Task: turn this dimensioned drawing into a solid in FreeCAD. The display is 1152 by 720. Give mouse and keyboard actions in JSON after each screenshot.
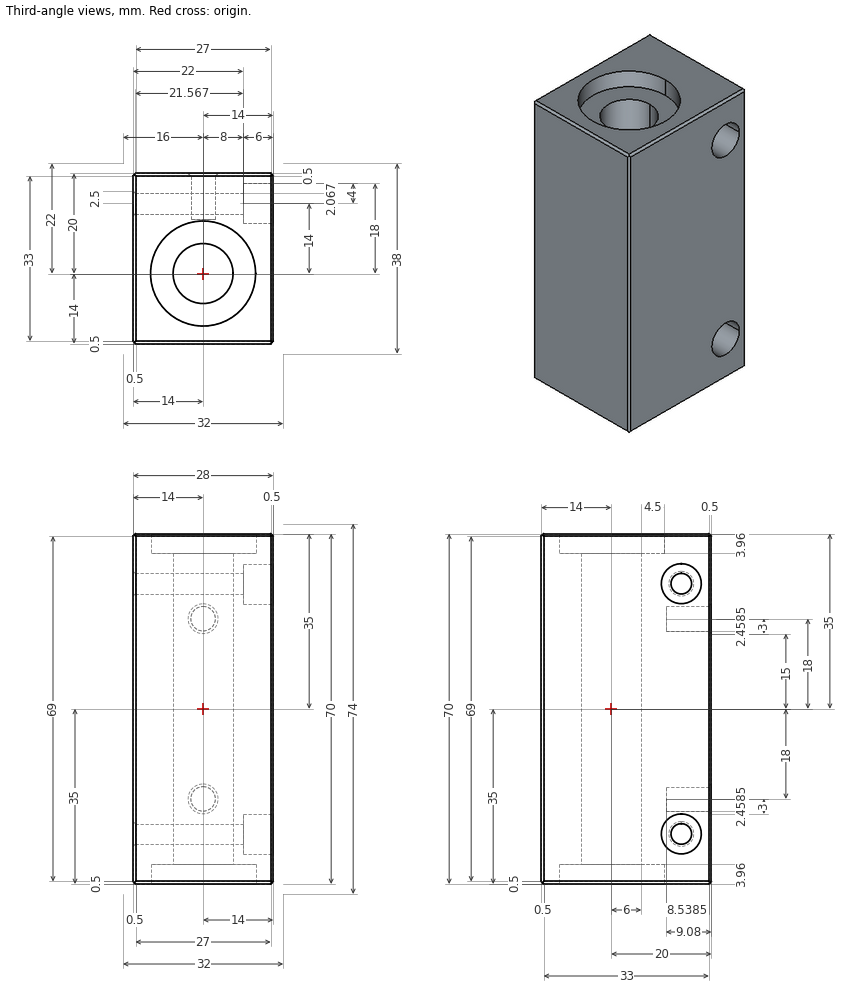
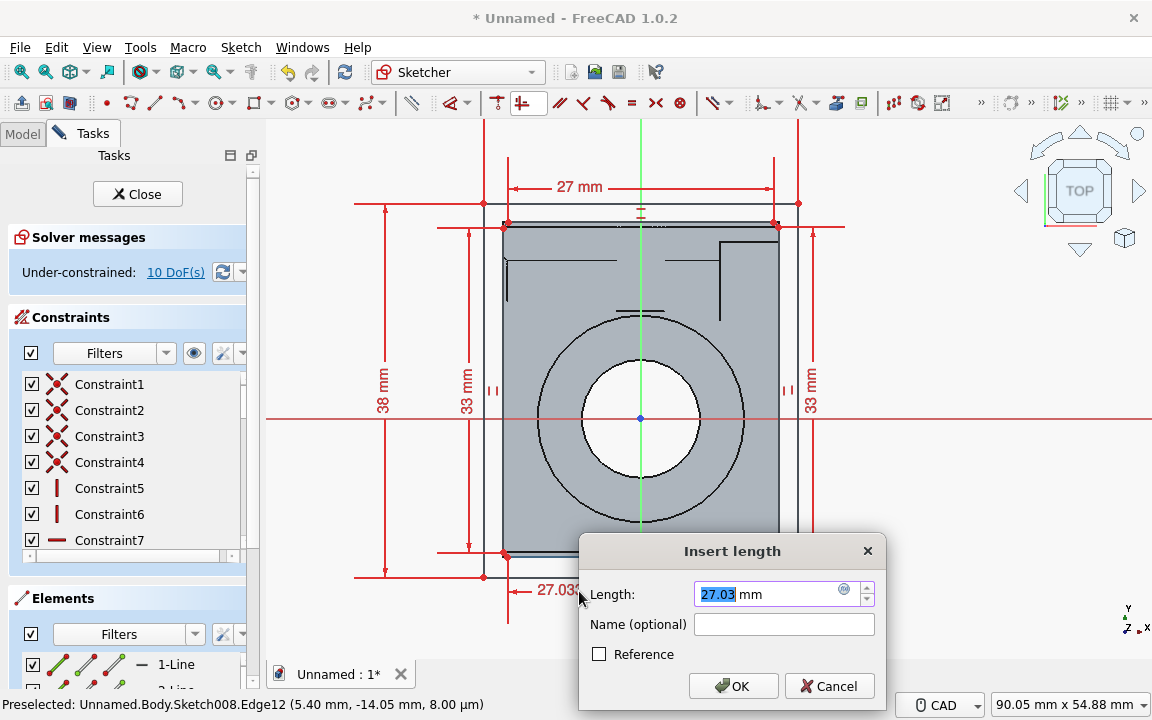
{"action": "type", "text": "27"}
{"action": "key", "text": "Return"}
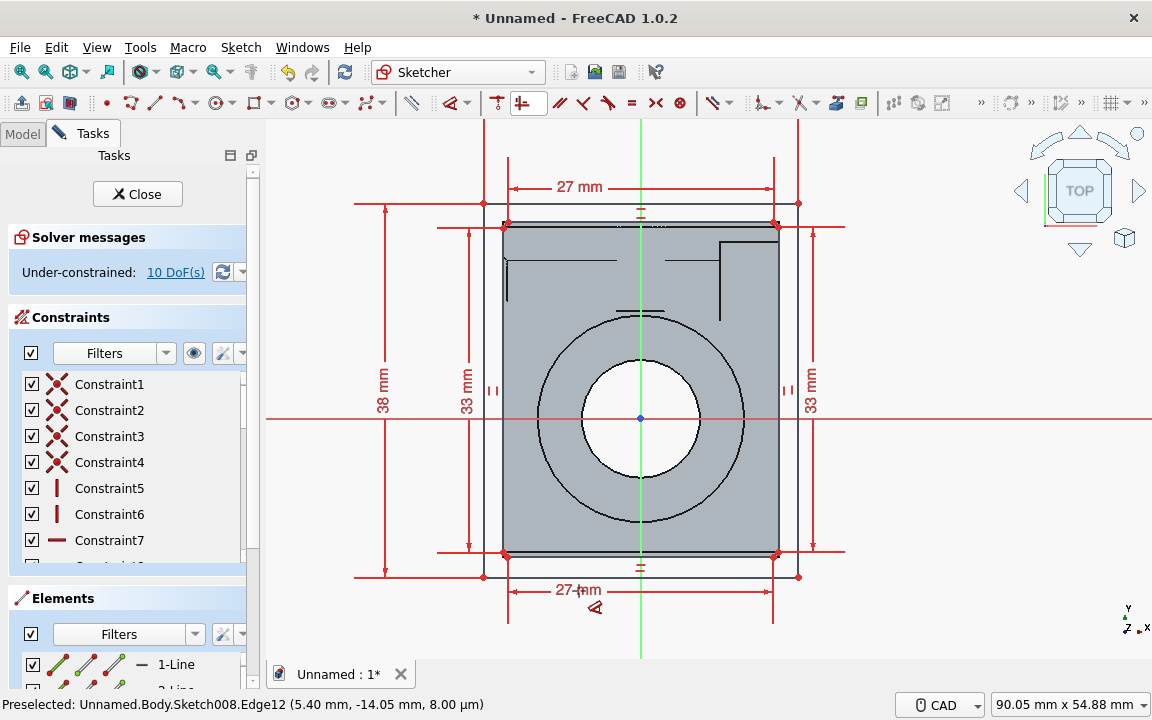
{"action": "left_click", "coordinate": [484, 204]}
{"action": "left_click", "coordinate": [507, 170]}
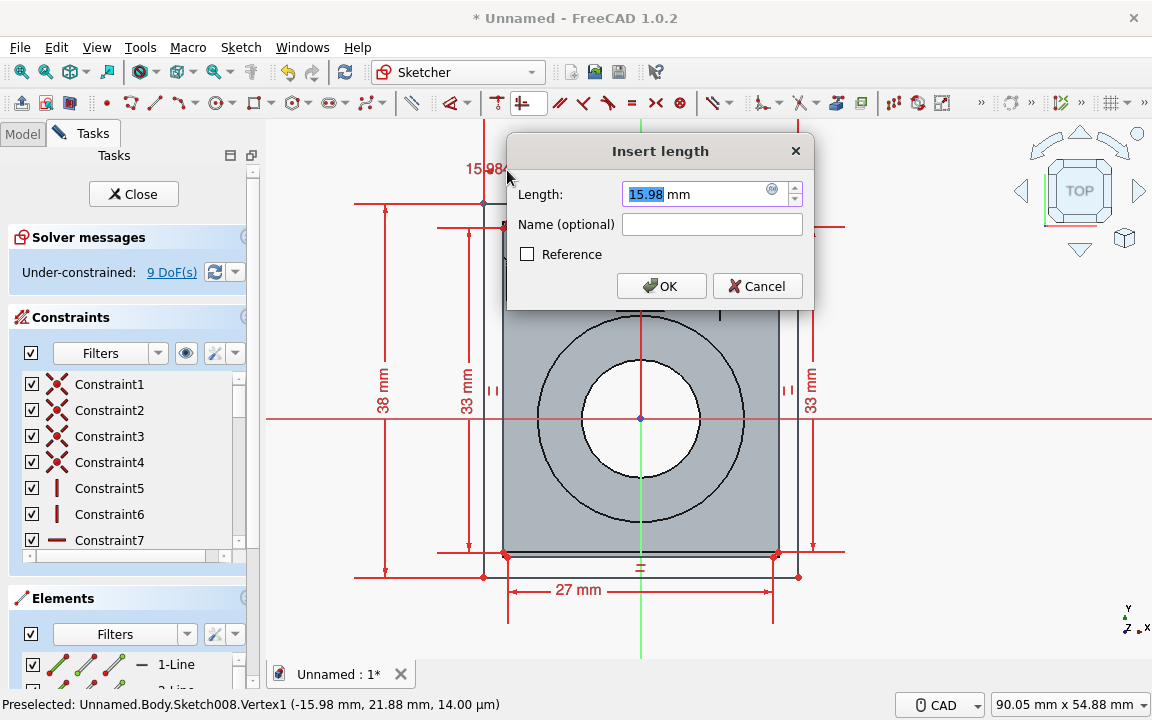
{"action": "type", "text": "16"}
{"action": "key", "text": "Return"}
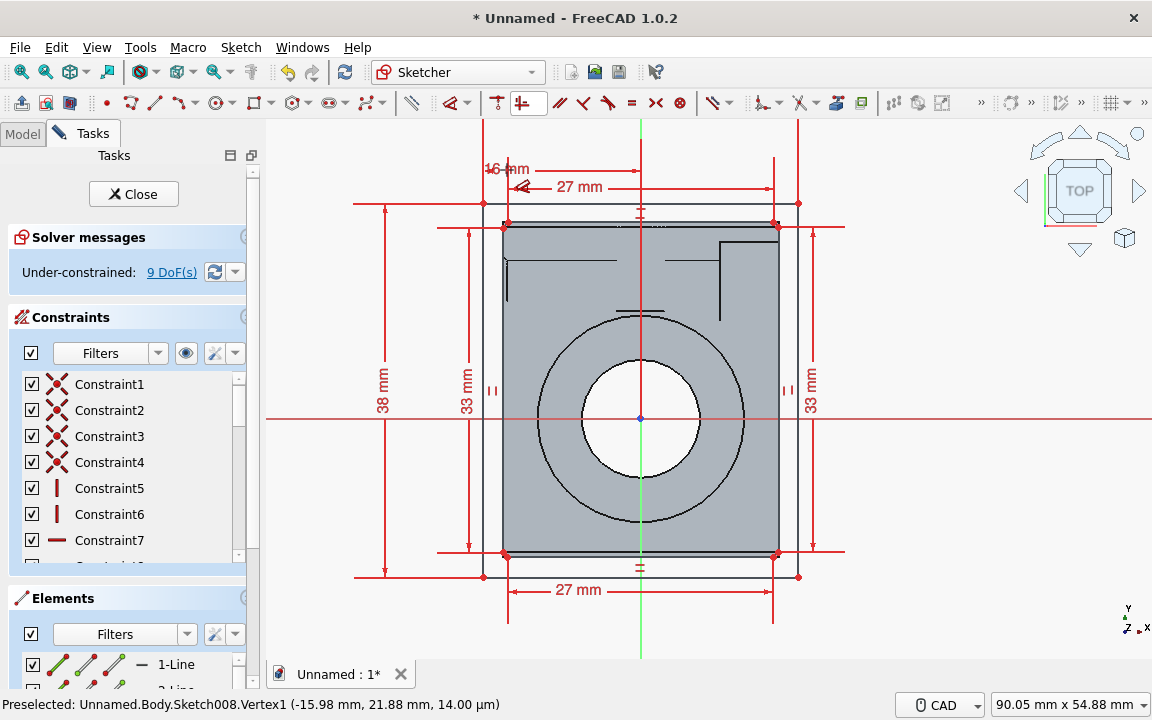
{"action": "left_click", "coordinate": [483, 204]}
{"action": "left_click", "coordinate": [449, 311]}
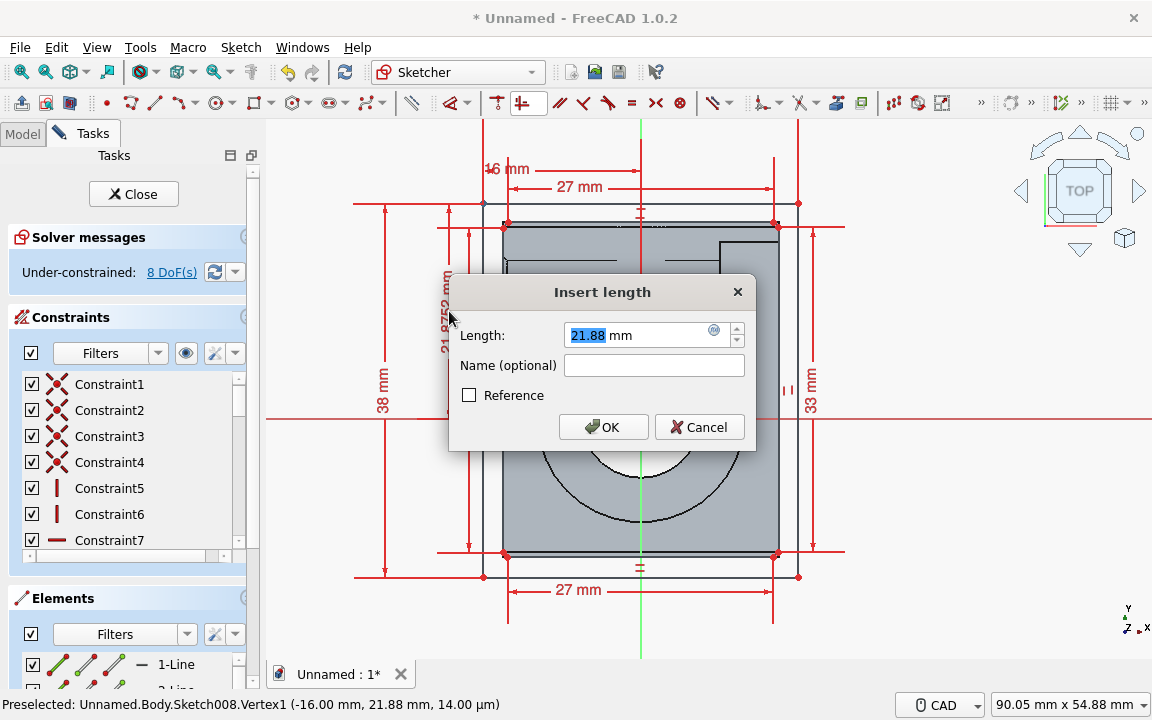
{"action": "type", "text": "22"}
{"action": "key", "text": "Return"}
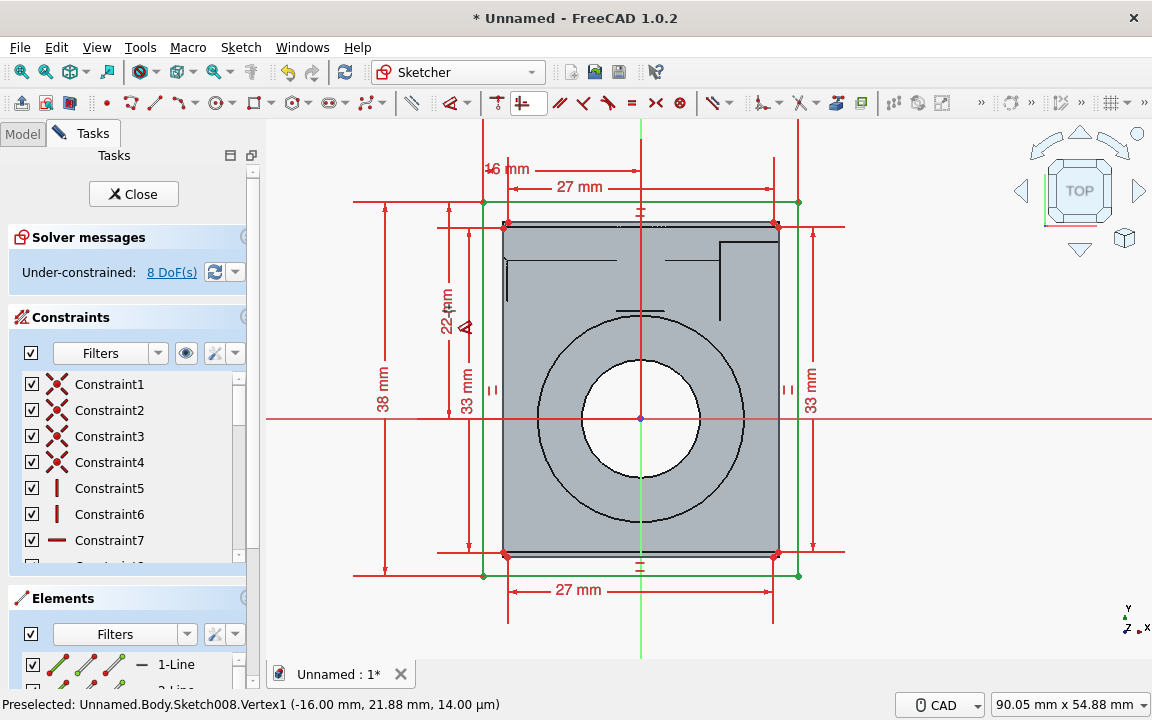
{"action": "scroll", "coordinate": [508, 557], "scroll_direction": "up", "scroll_amount": 4}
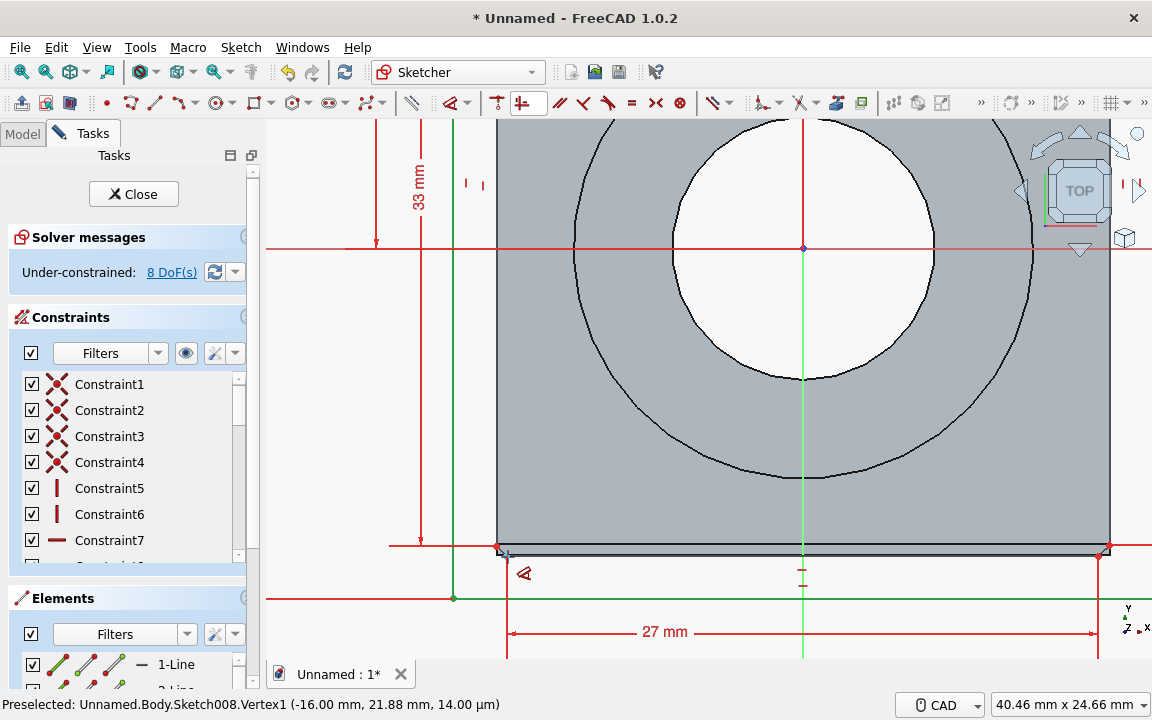
{"action": "left_click", "coordinate": [507, 556]}
{"action": "left_click", "coordinate": [473, 402]}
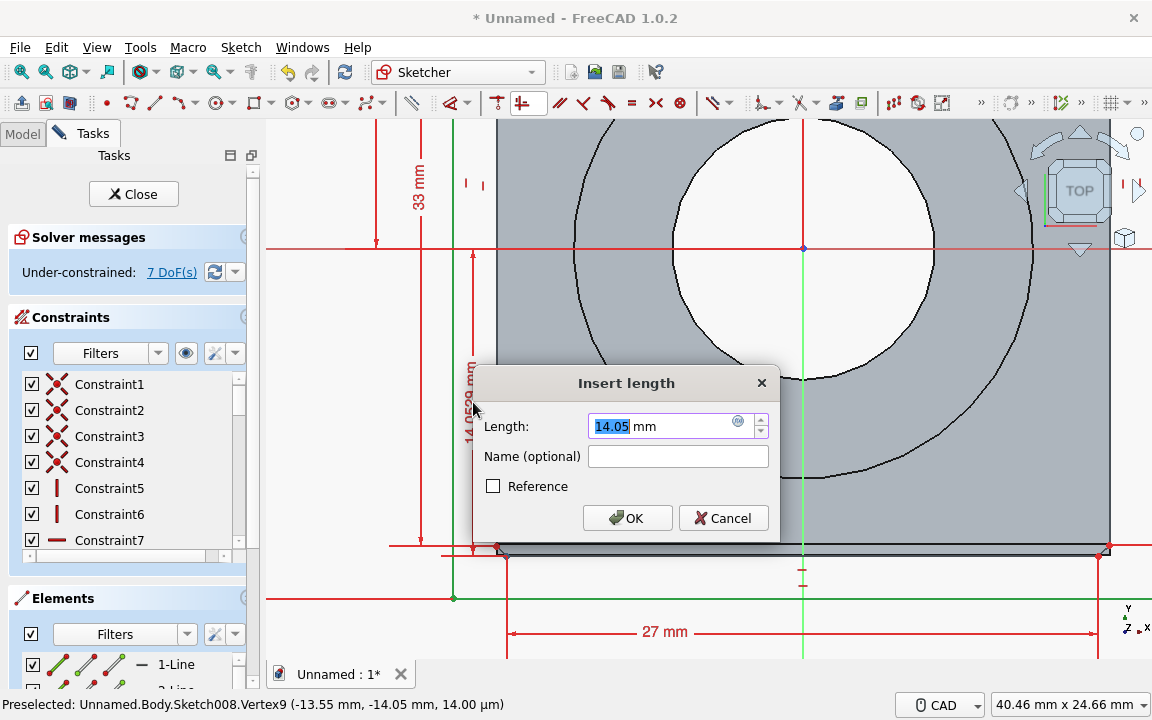
{"action": "type", "text": "14"}
{"action": "key", "text": "Return"}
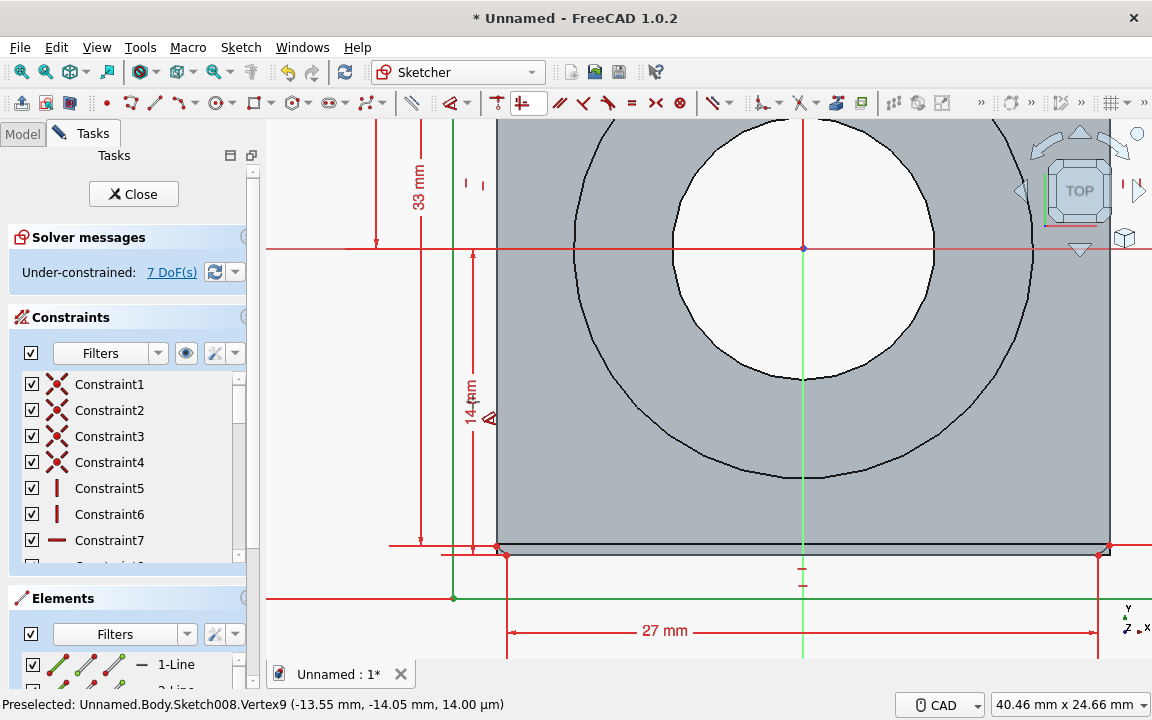
{"action": "left_click", "coordinate": [497, 546]}
{"action": "left_click", "coordinate": [650, 580]}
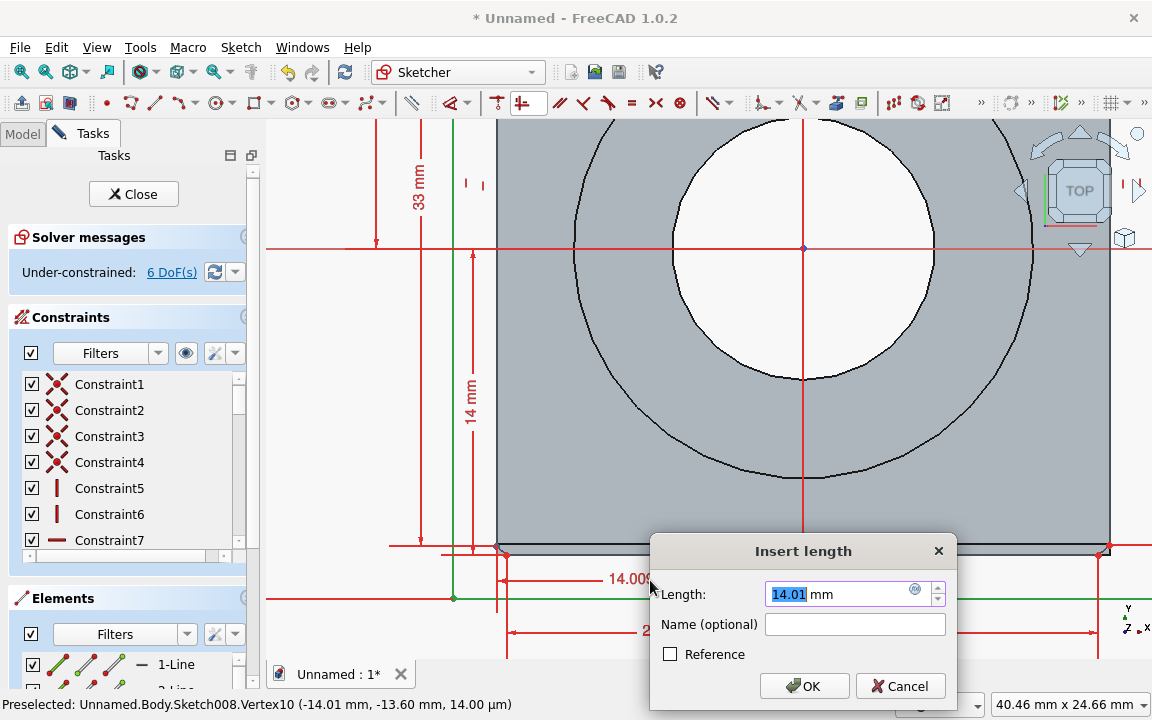
{"action": "type", "text": "14"}
{"action": "key", "text": "Return"}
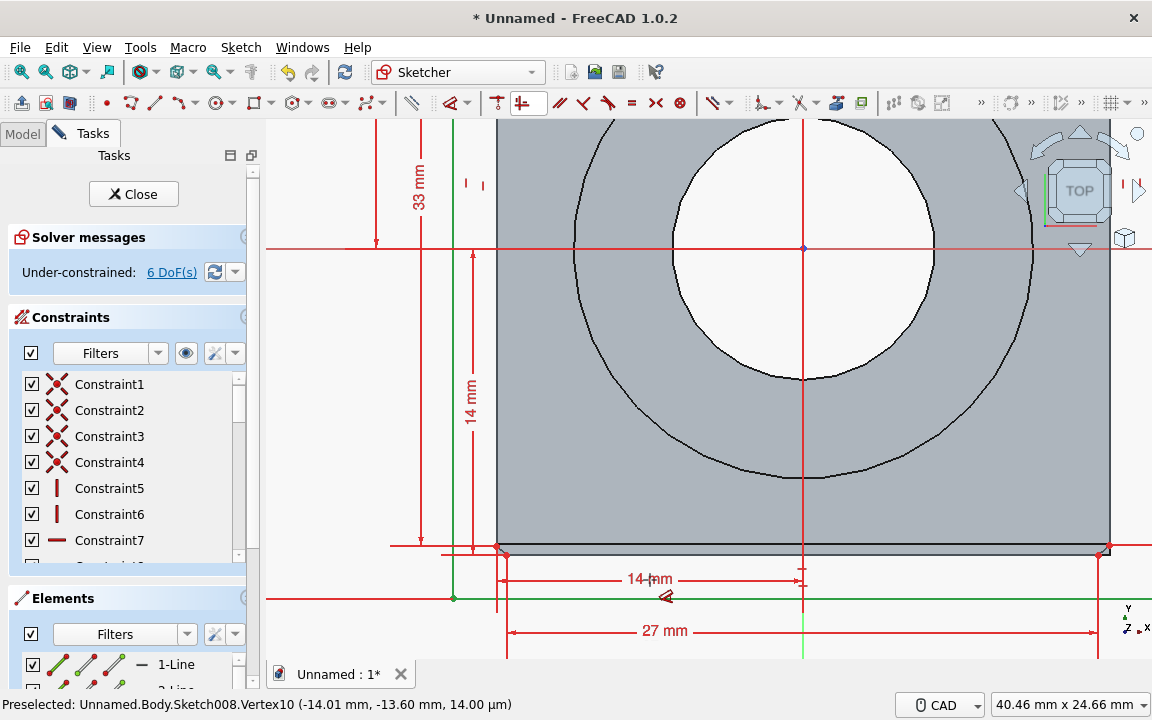
{"action": "scroll", "coordinate": [508, 557], "scroll_direction": "down", "scroll_amount": 4}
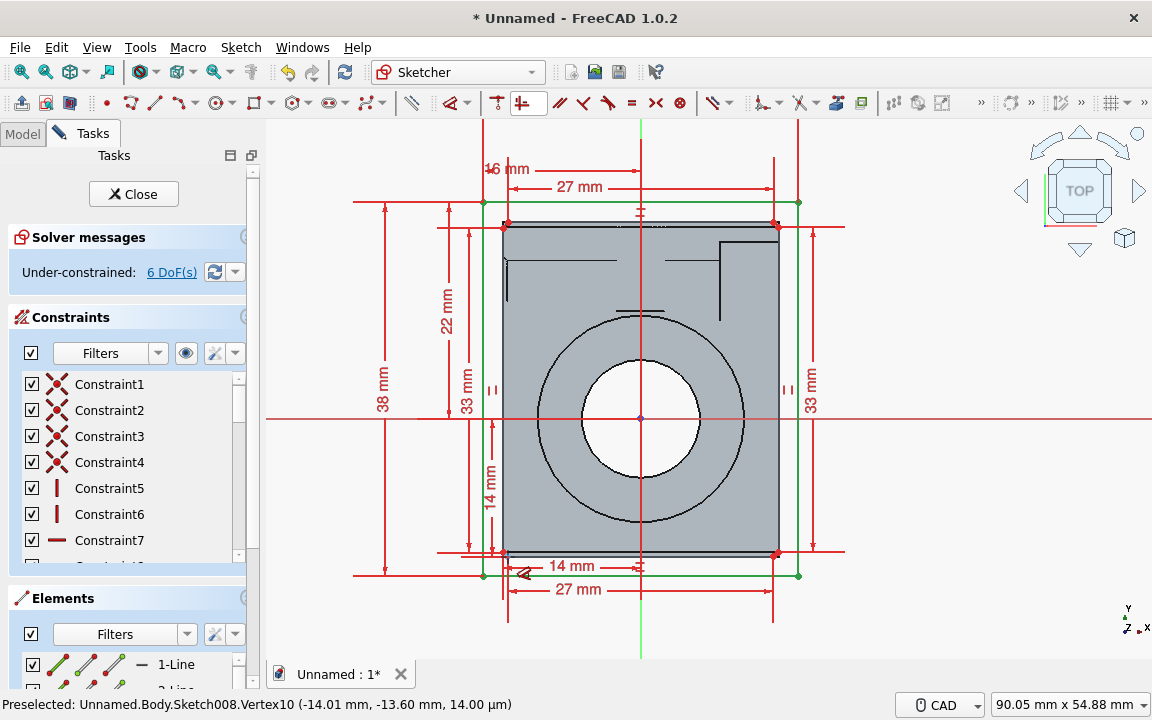
{"action": "scroll", "coordinate": [508, 222], "scroll_direction": "up", "scroll_amount": 3}